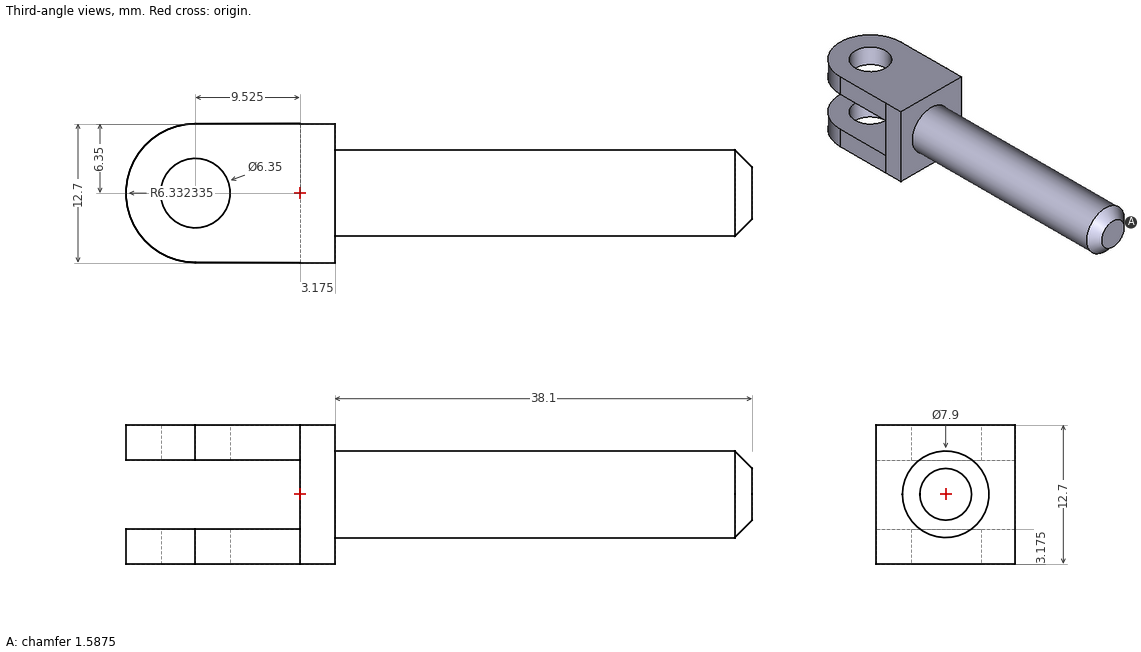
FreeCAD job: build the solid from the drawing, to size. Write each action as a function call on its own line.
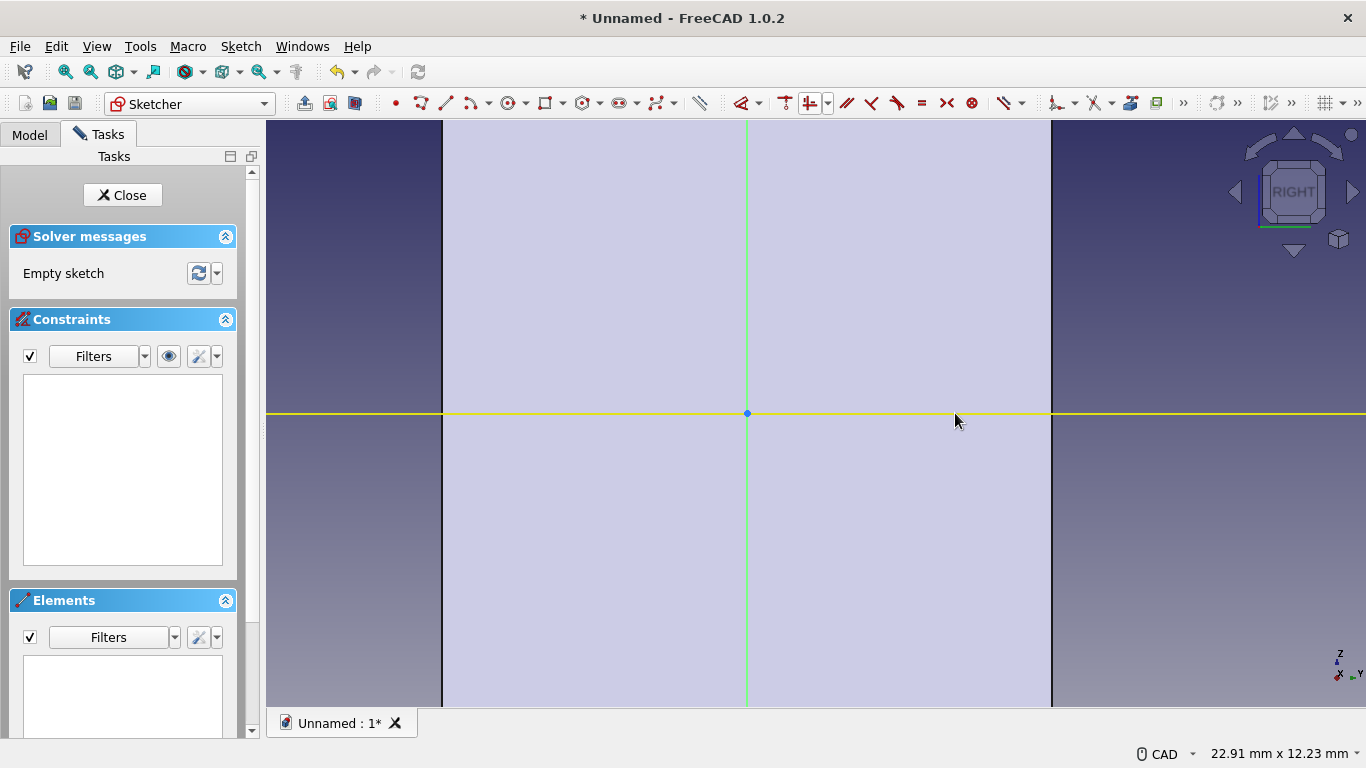
click(508, 104)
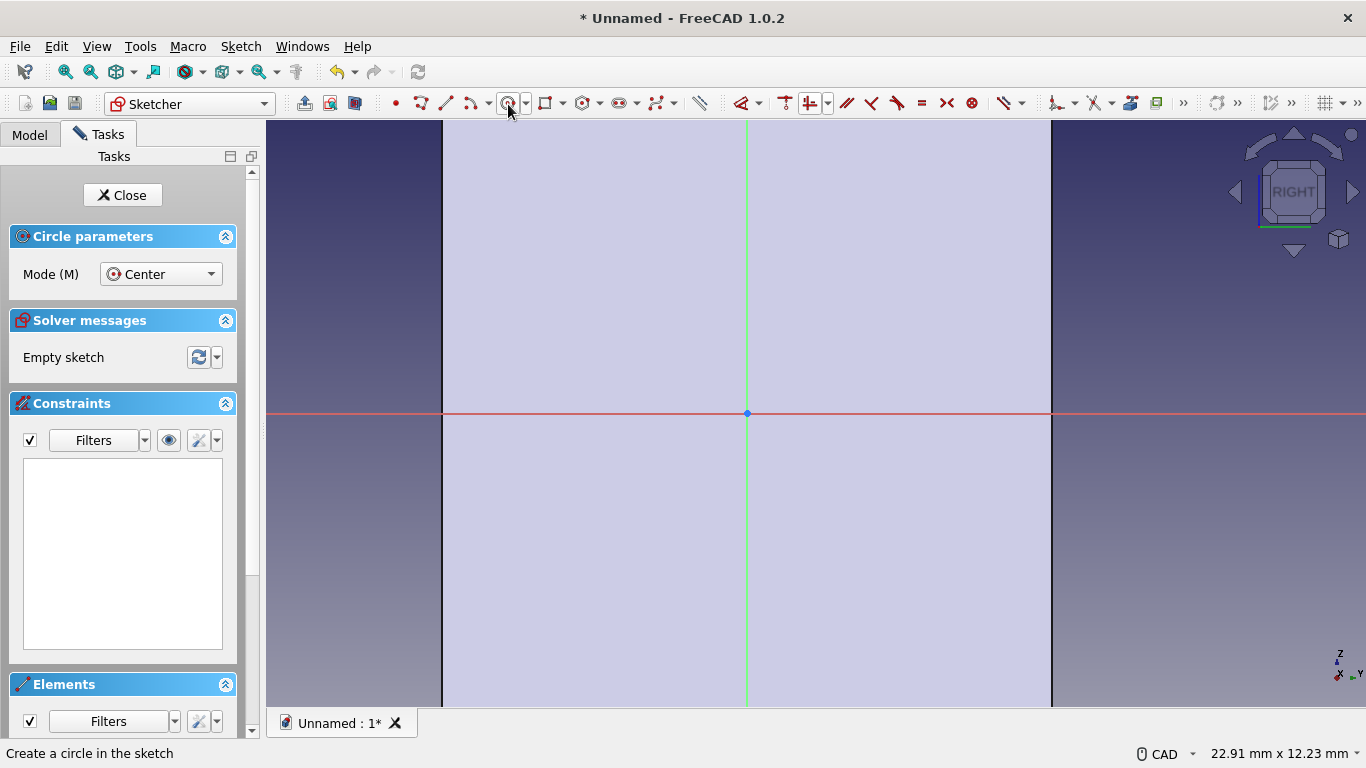
click(747, 414)
move(881, 279)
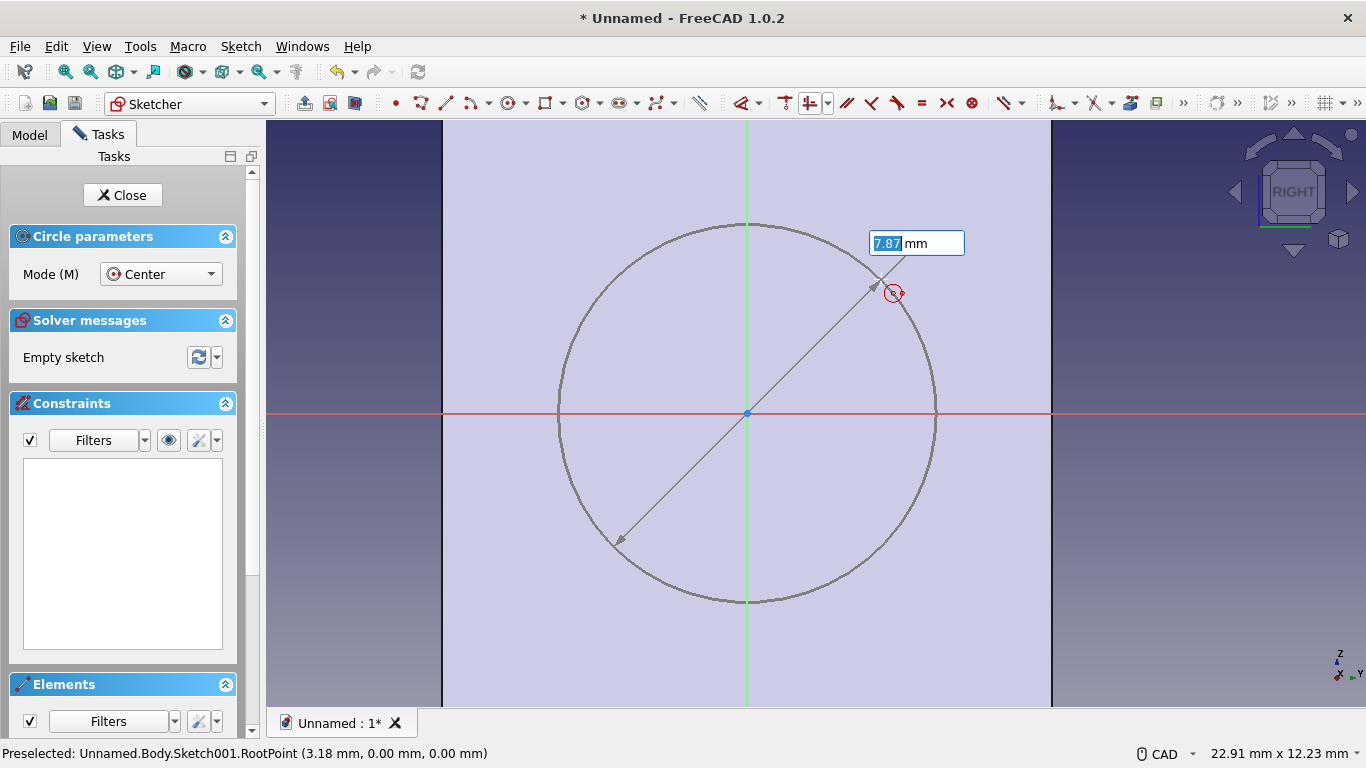
text(7.9)
key(Return)
key(Escape)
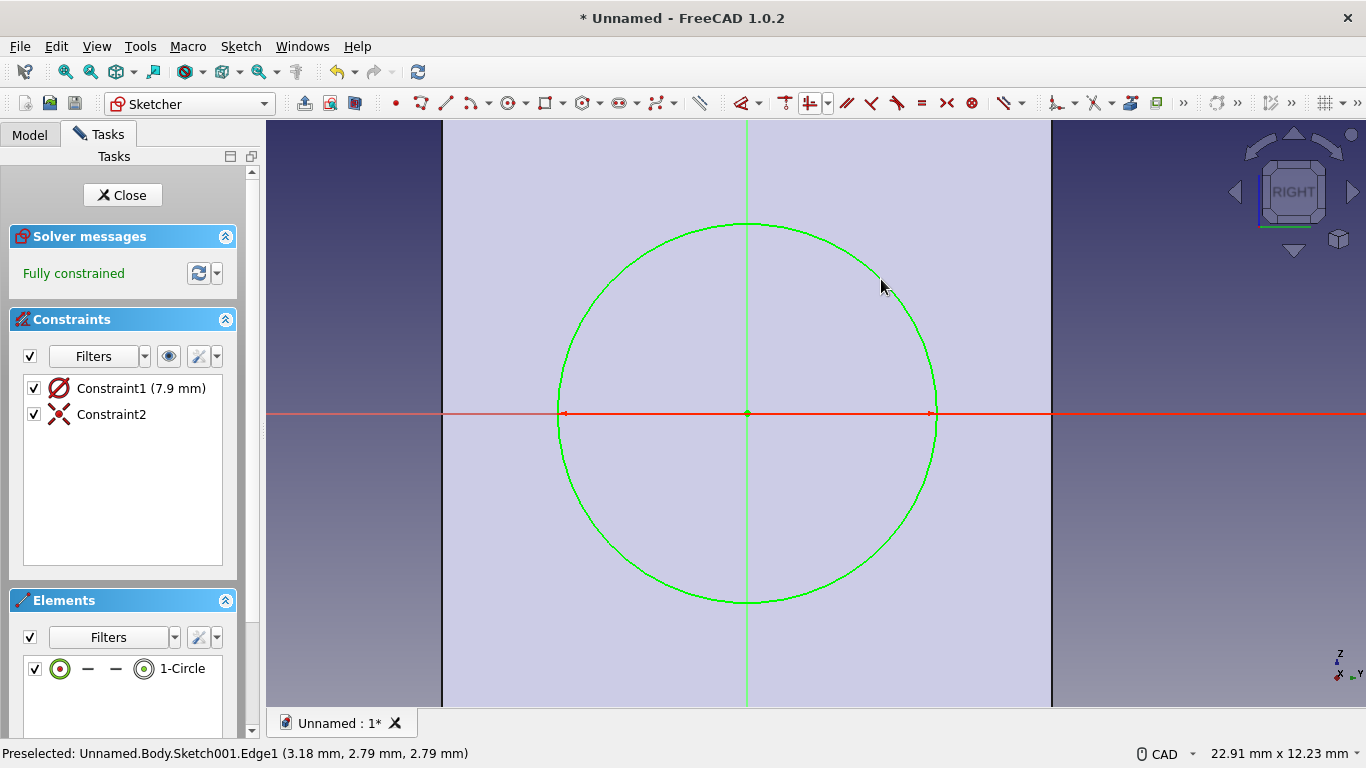
click(123, 195)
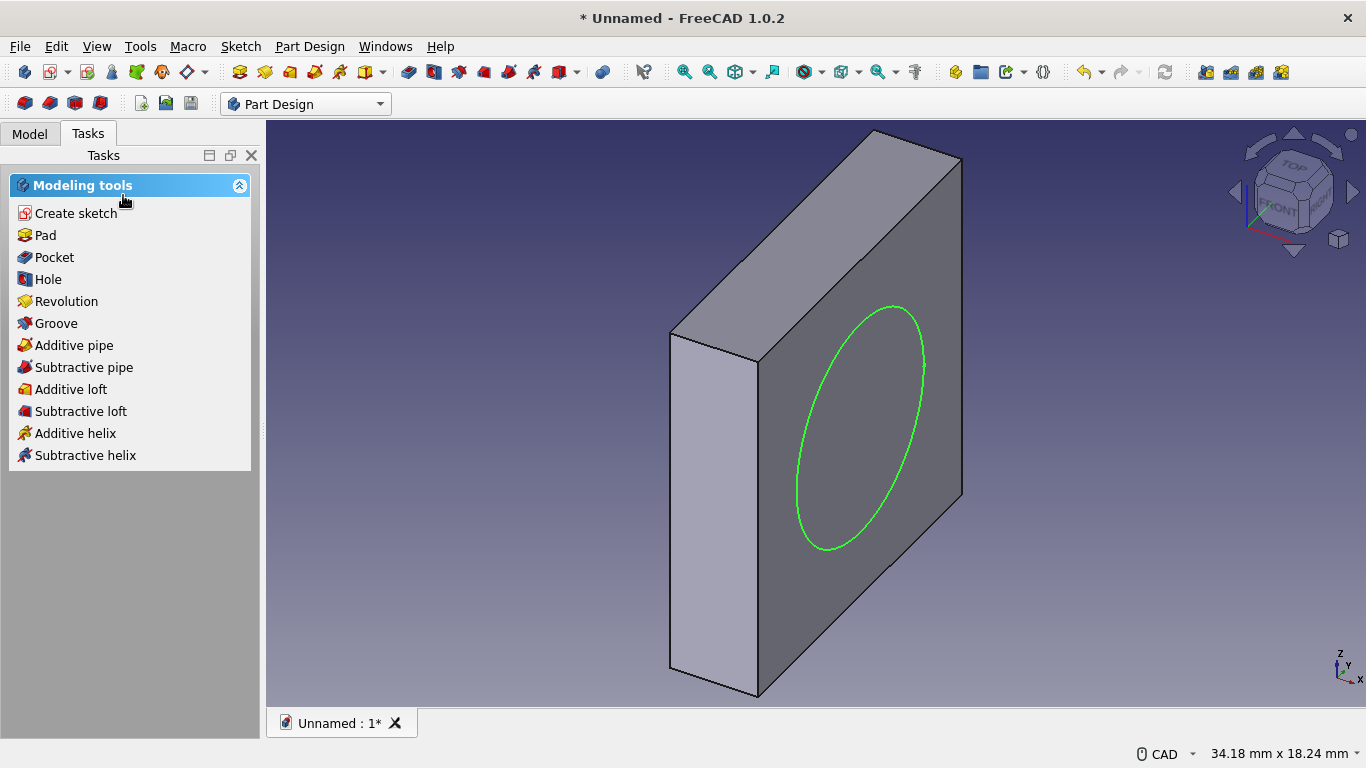
click(240, 72)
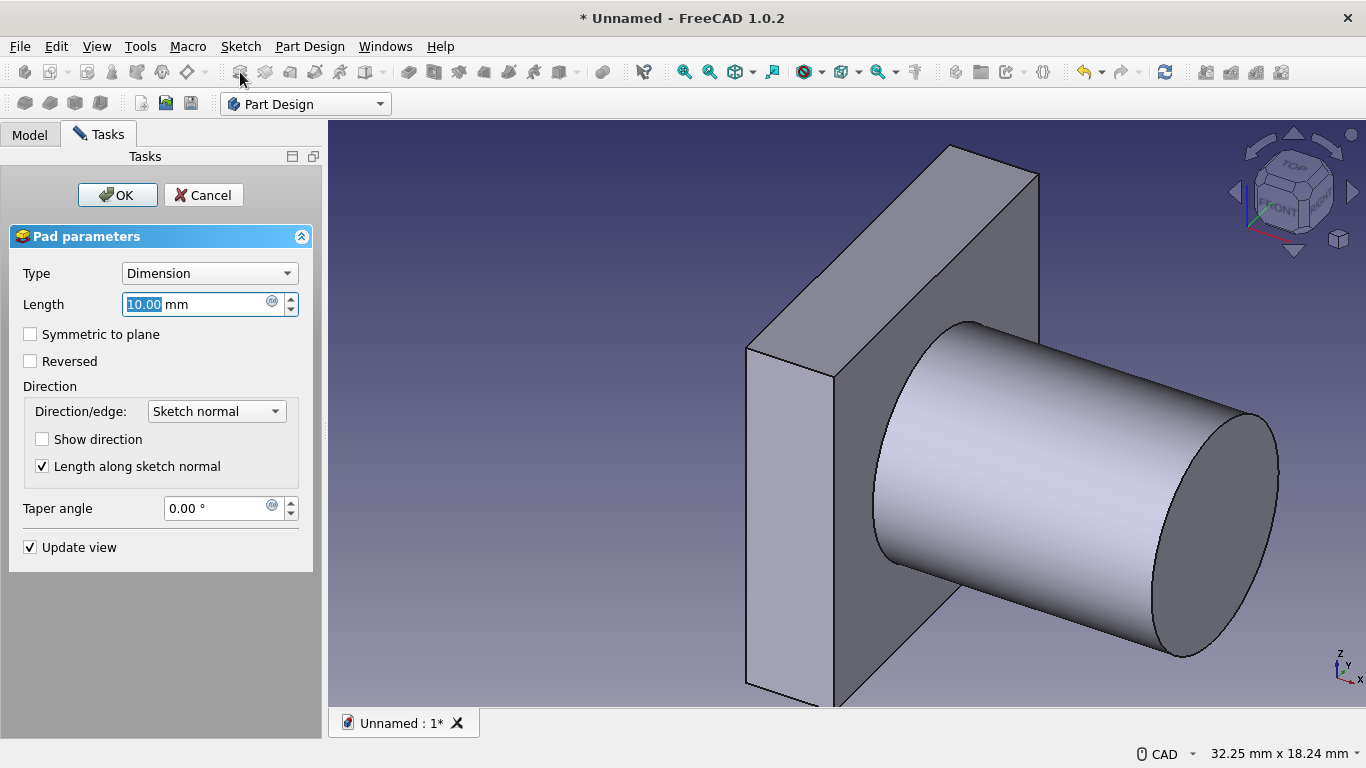
text(38.1)
key(Tab)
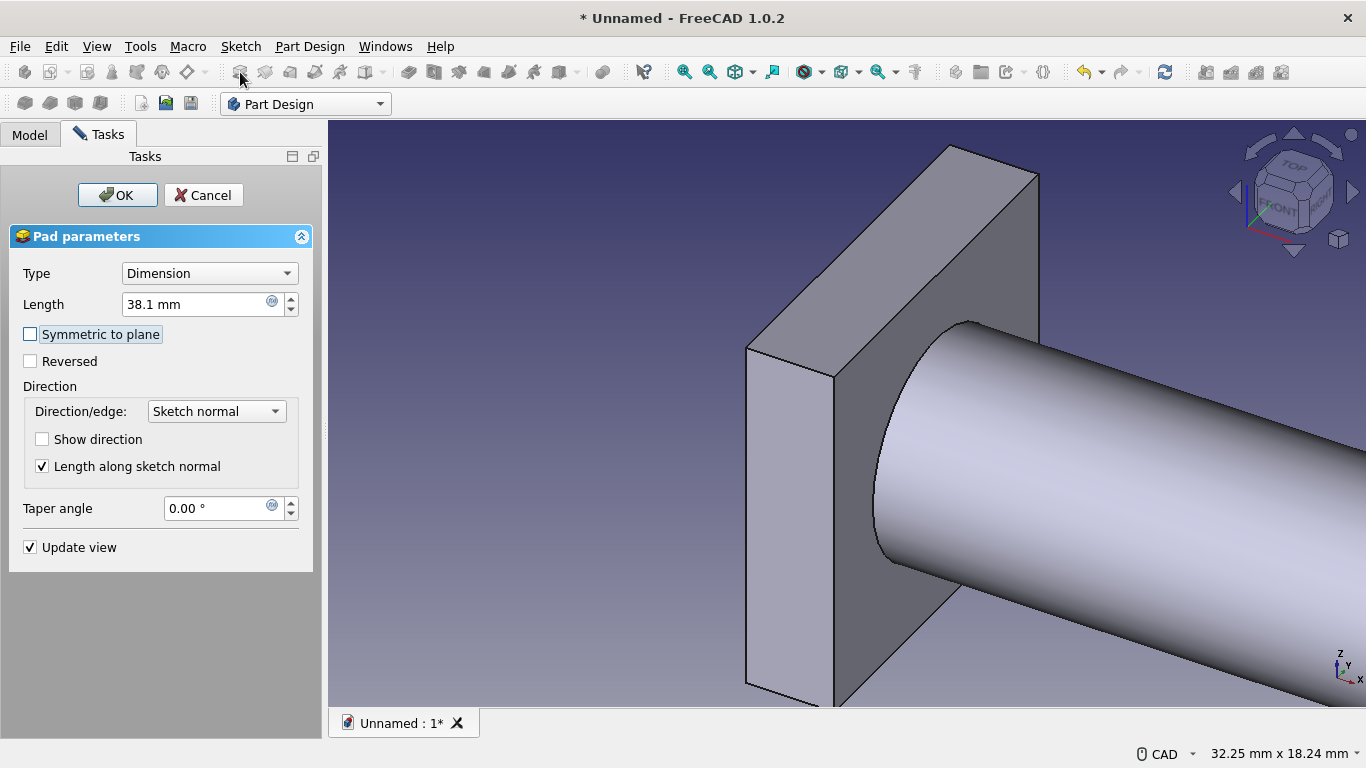
click(118, 195)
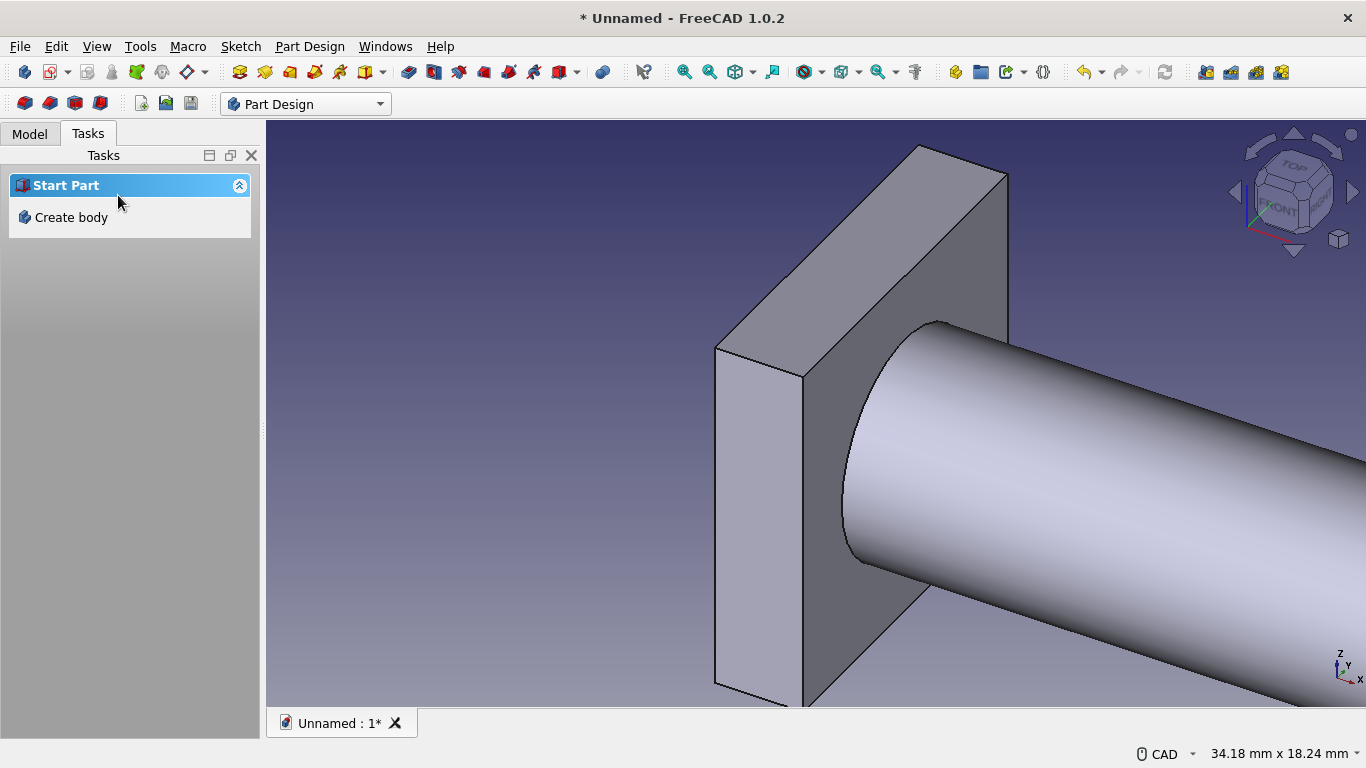
click(685, 72)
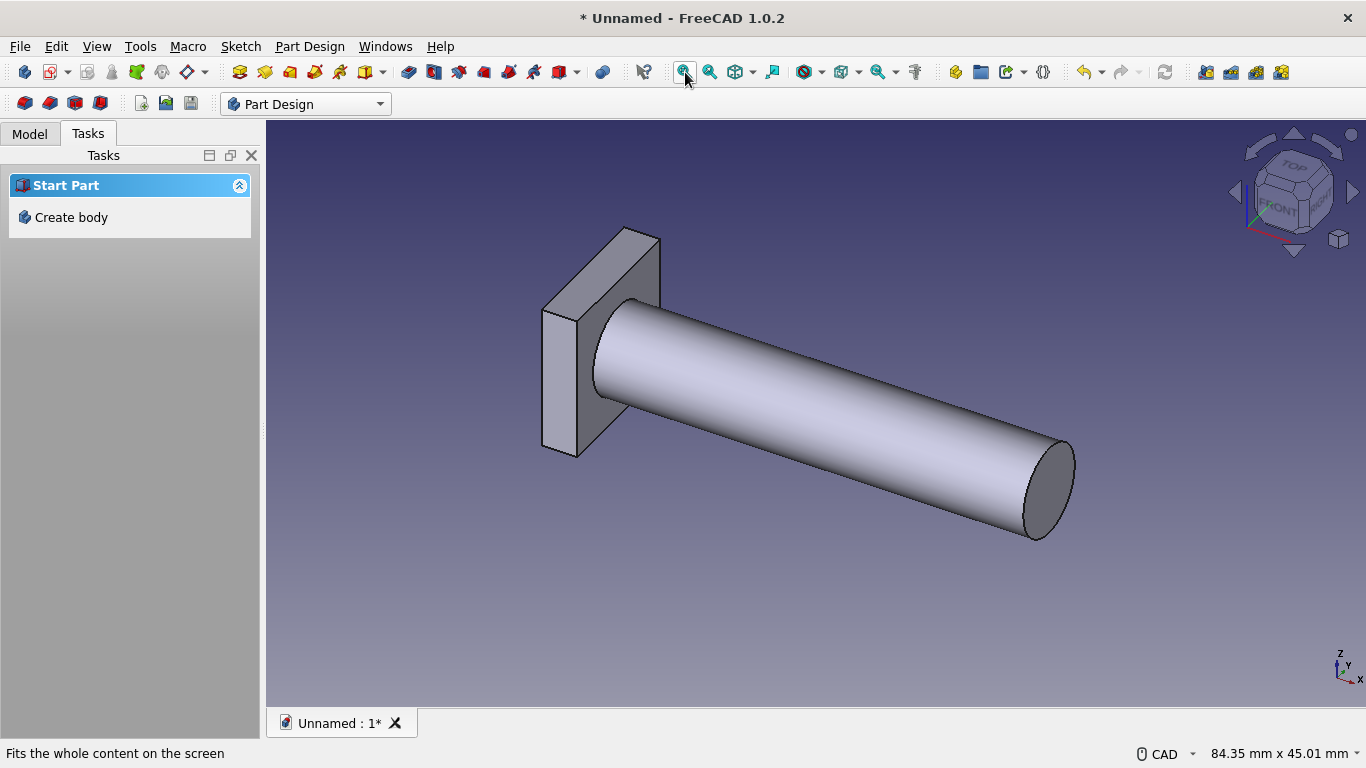
click(1023, 515)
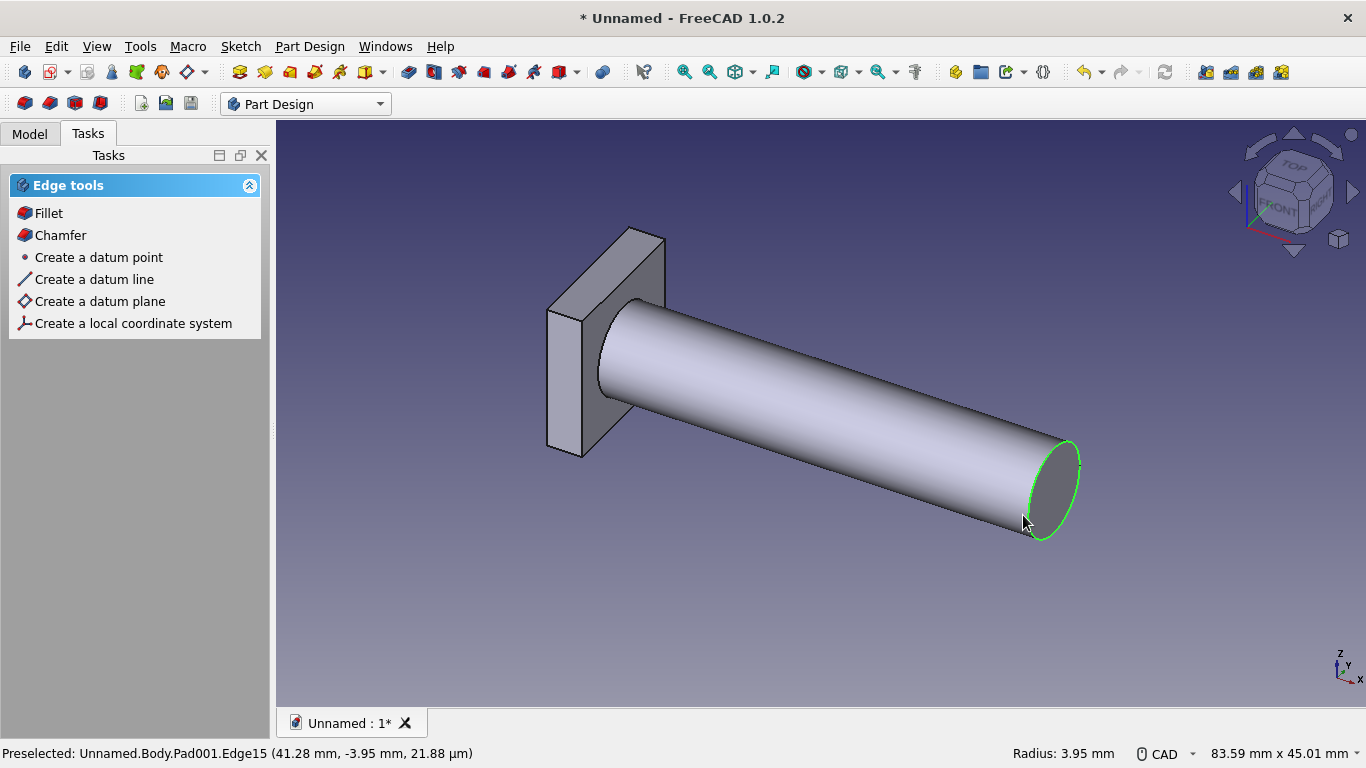
click(50, 104)